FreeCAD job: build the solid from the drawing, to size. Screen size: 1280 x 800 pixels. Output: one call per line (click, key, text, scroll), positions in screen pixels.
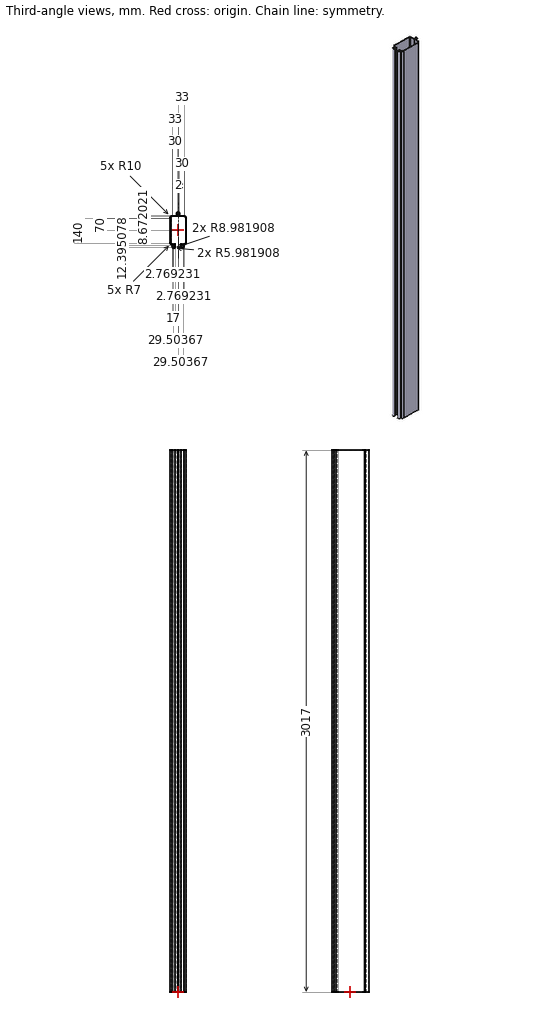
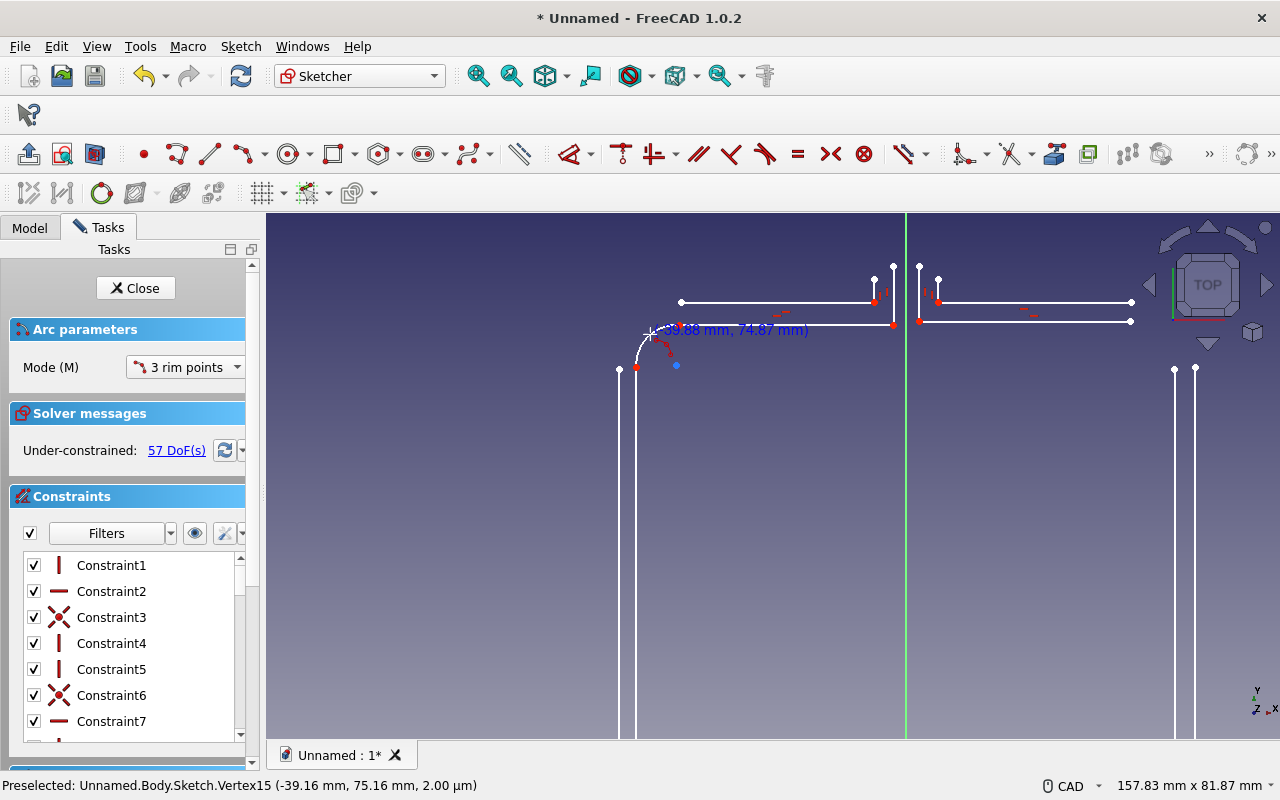
scroll(893, 266, up, 2)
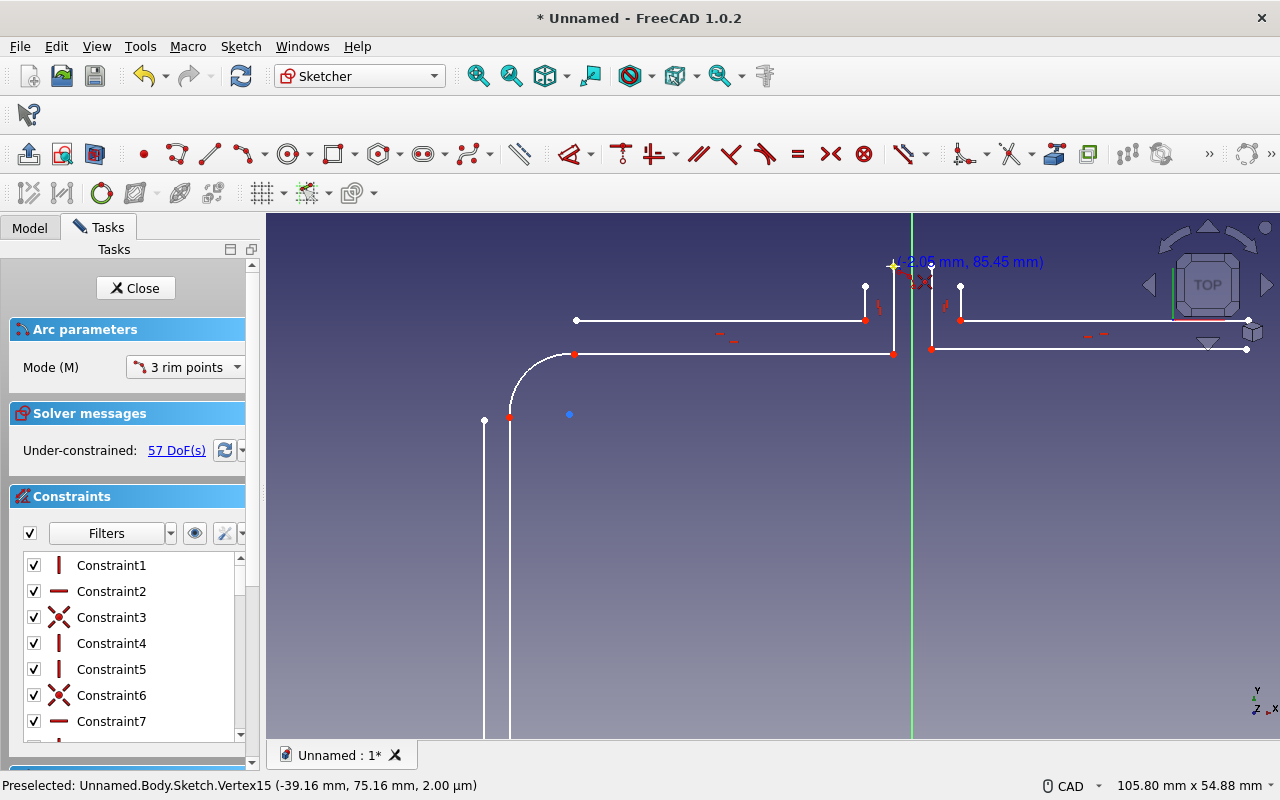
click(894, 266)
click(932, 266)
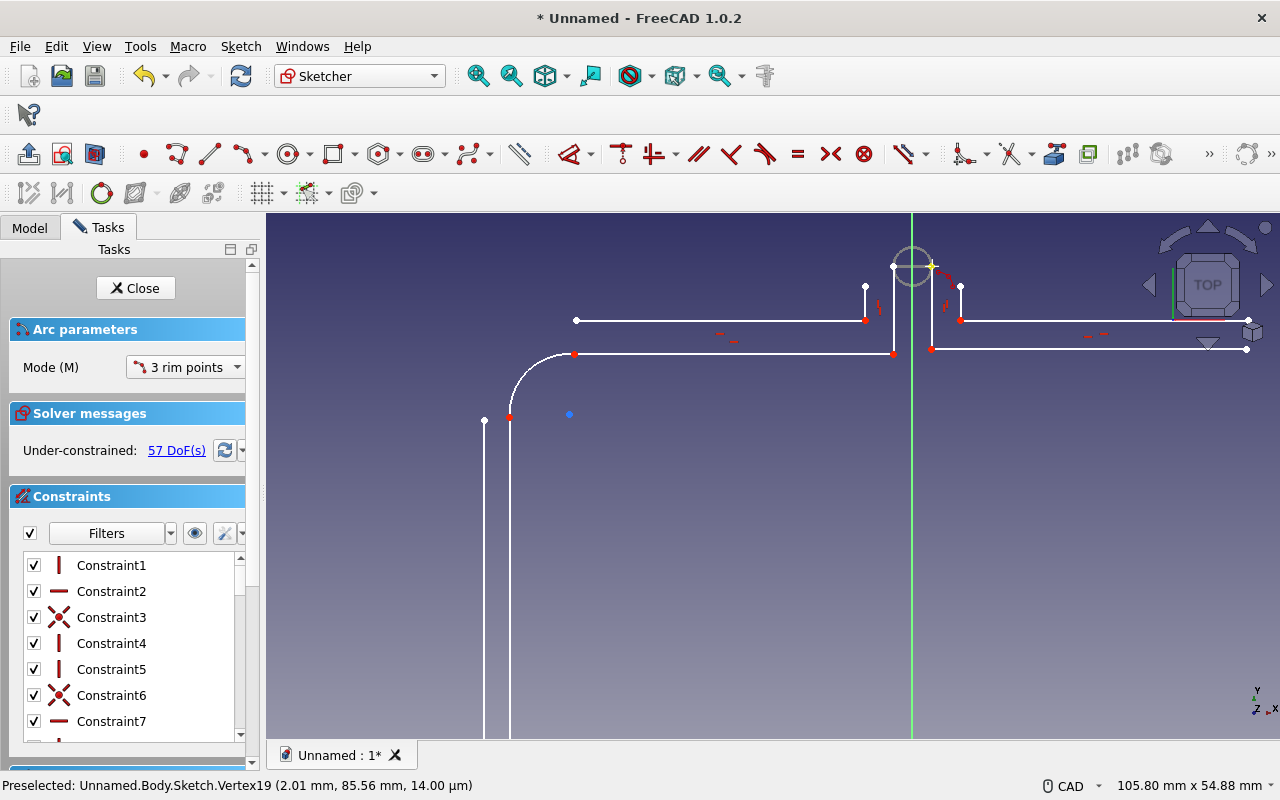
scroll(663, 356, down, 9)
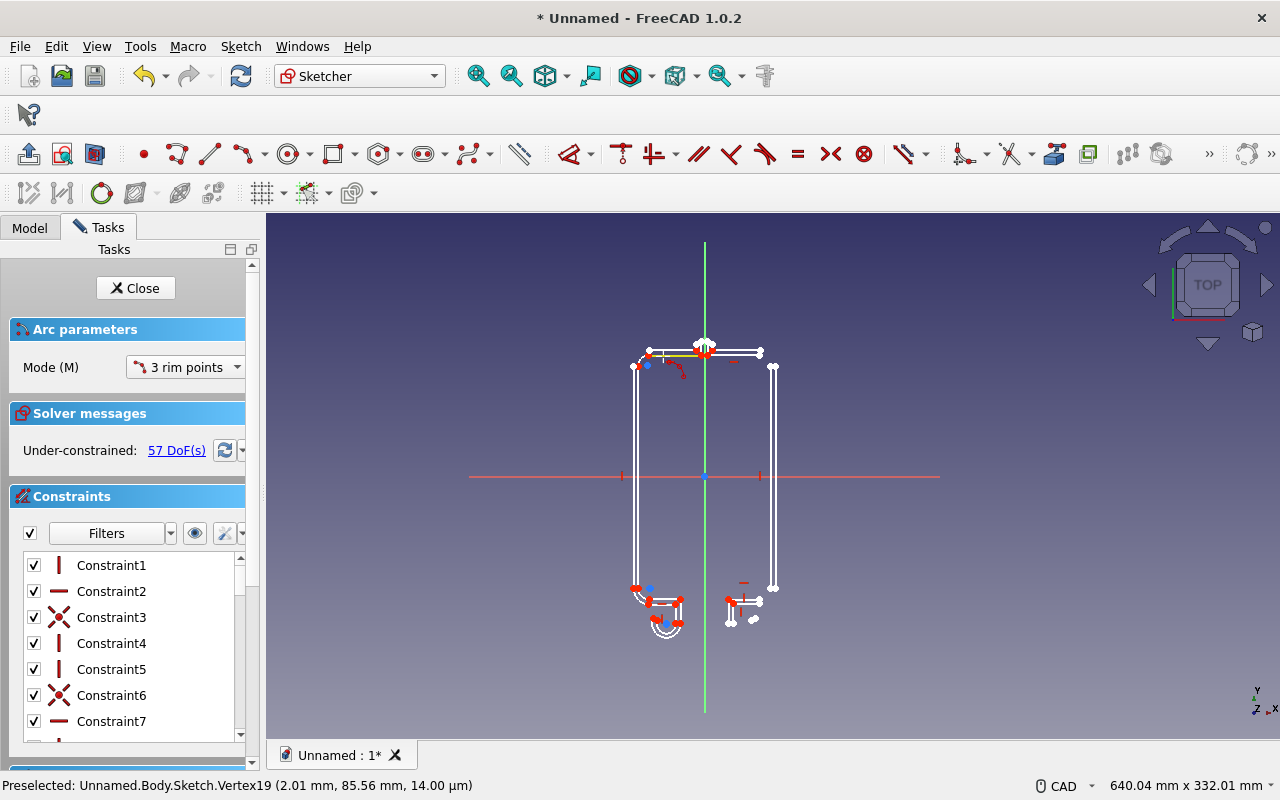
scroll(715, 326, up, 3)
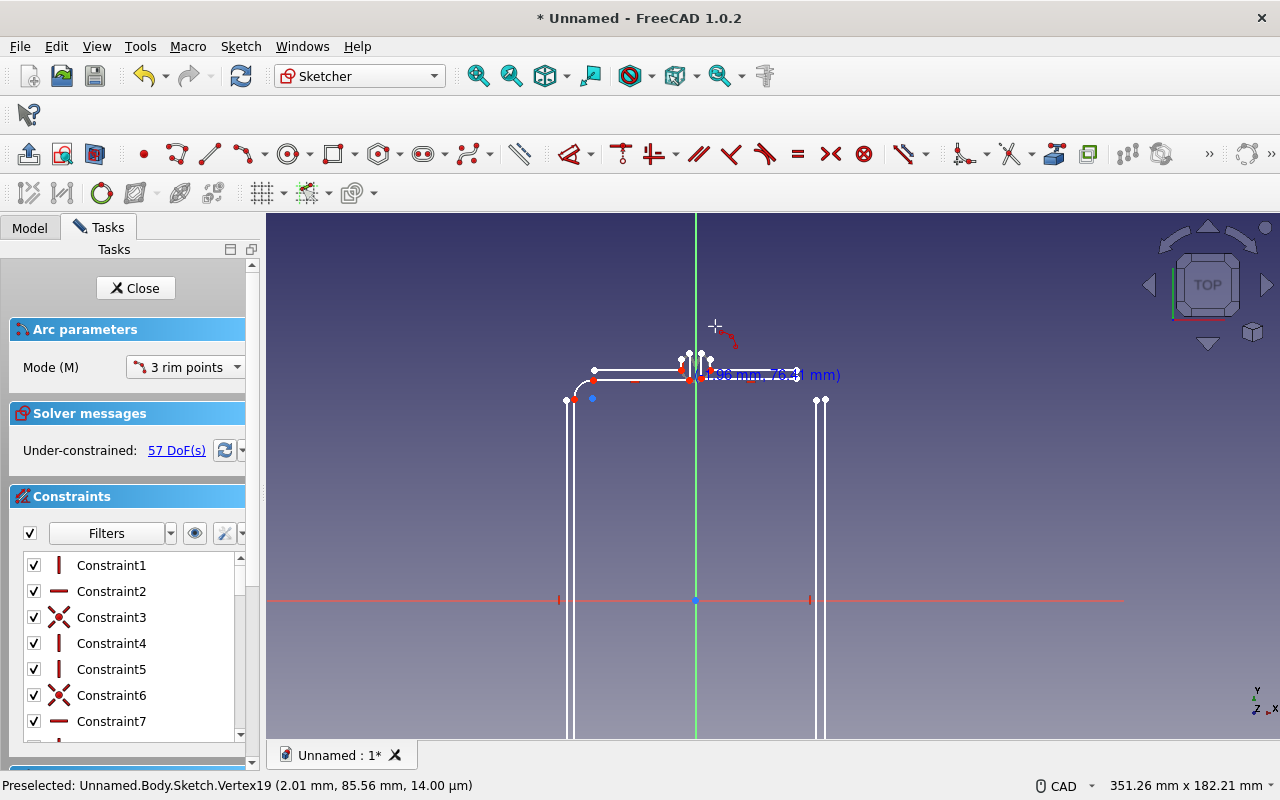
click(714, 326)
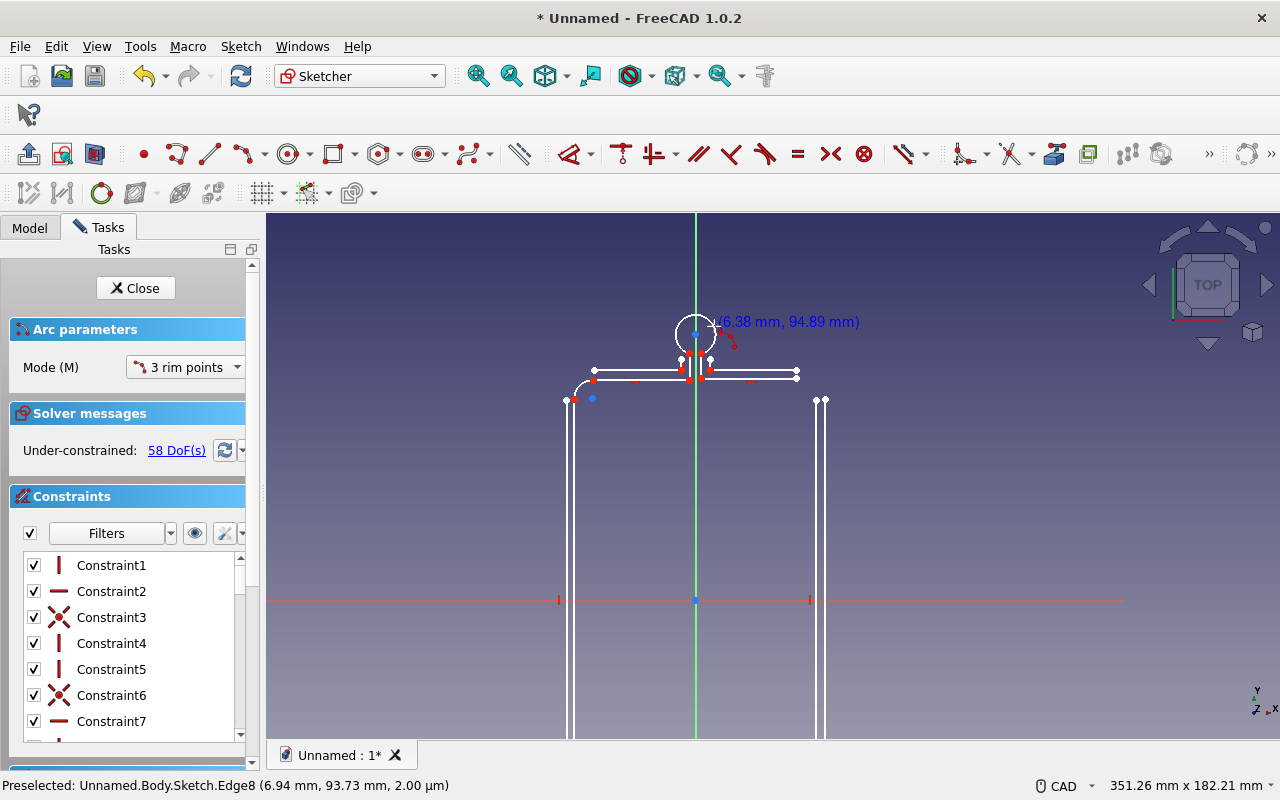
scroll(797, 379, up, 4)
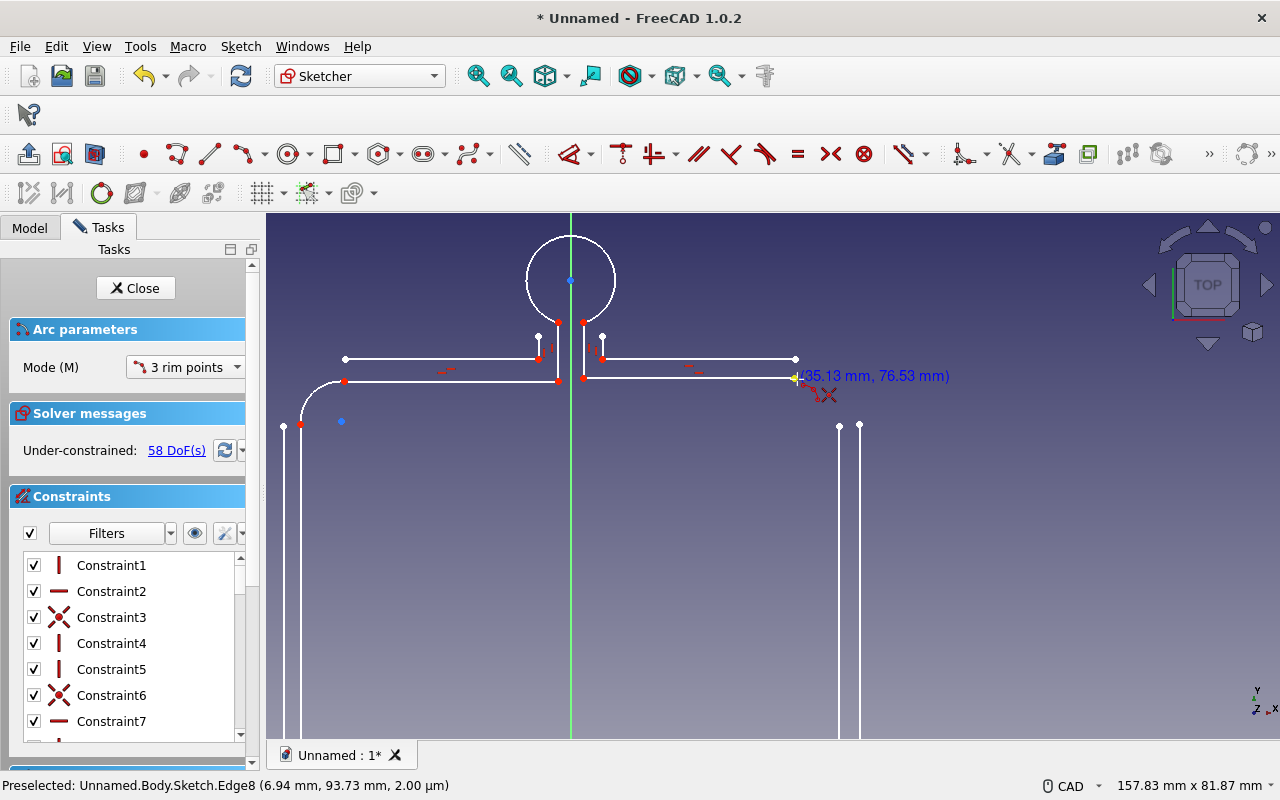
click(795, 378)
click(839, 426)
click(827, 391)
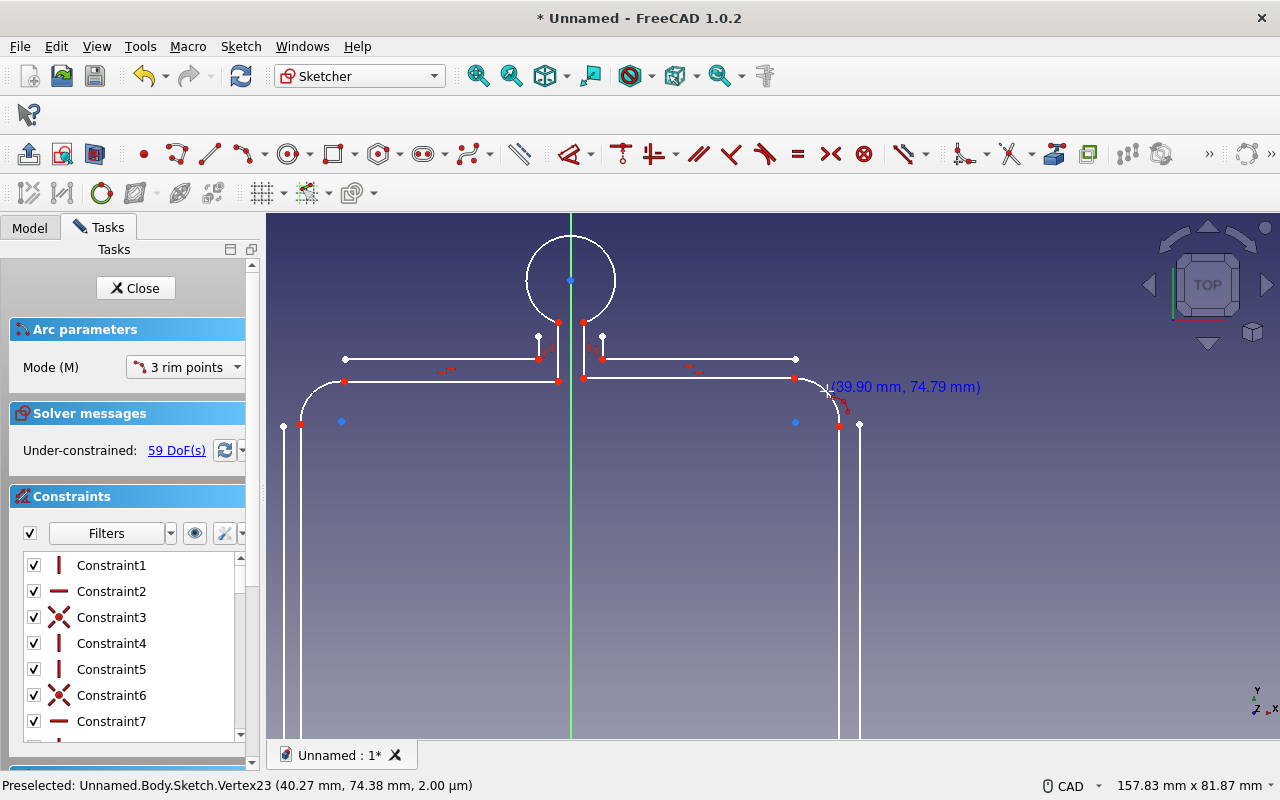
scroll(748, 347, down, 7)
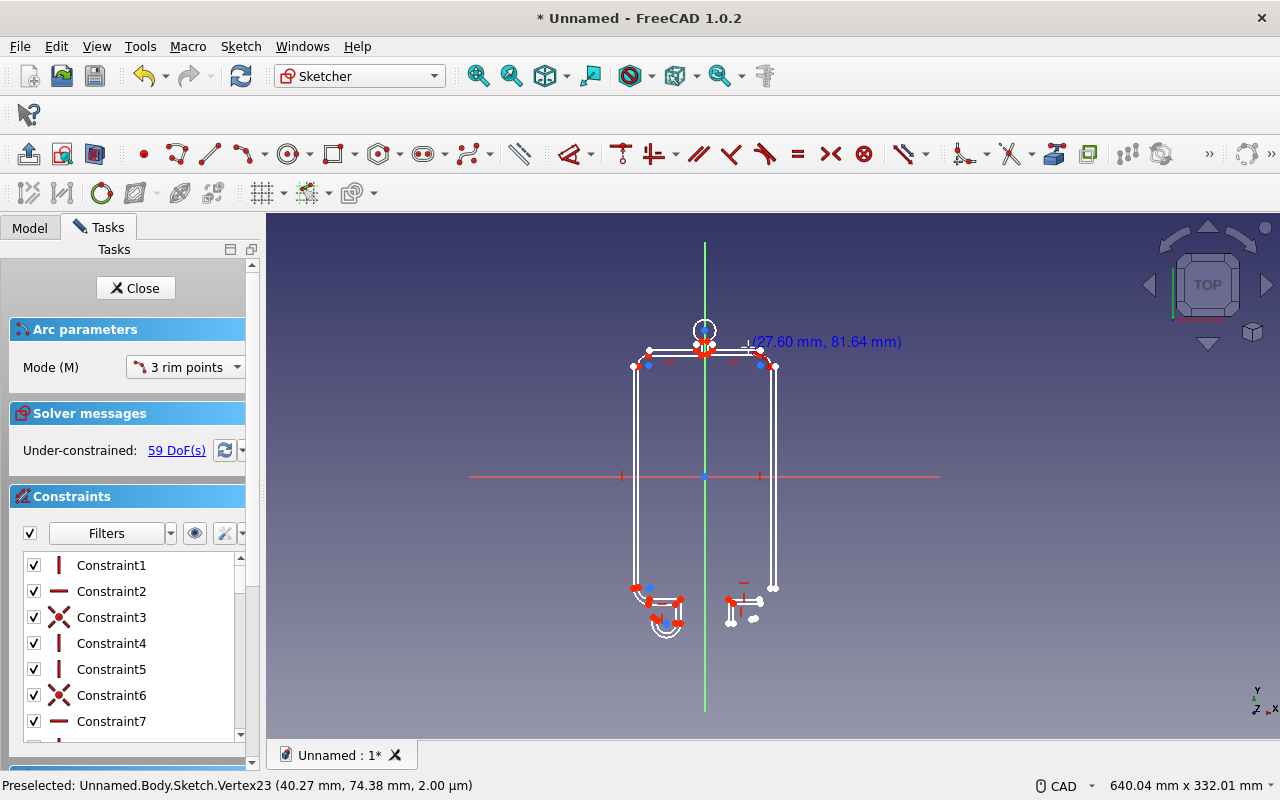
scroll(771, 588, up, 7)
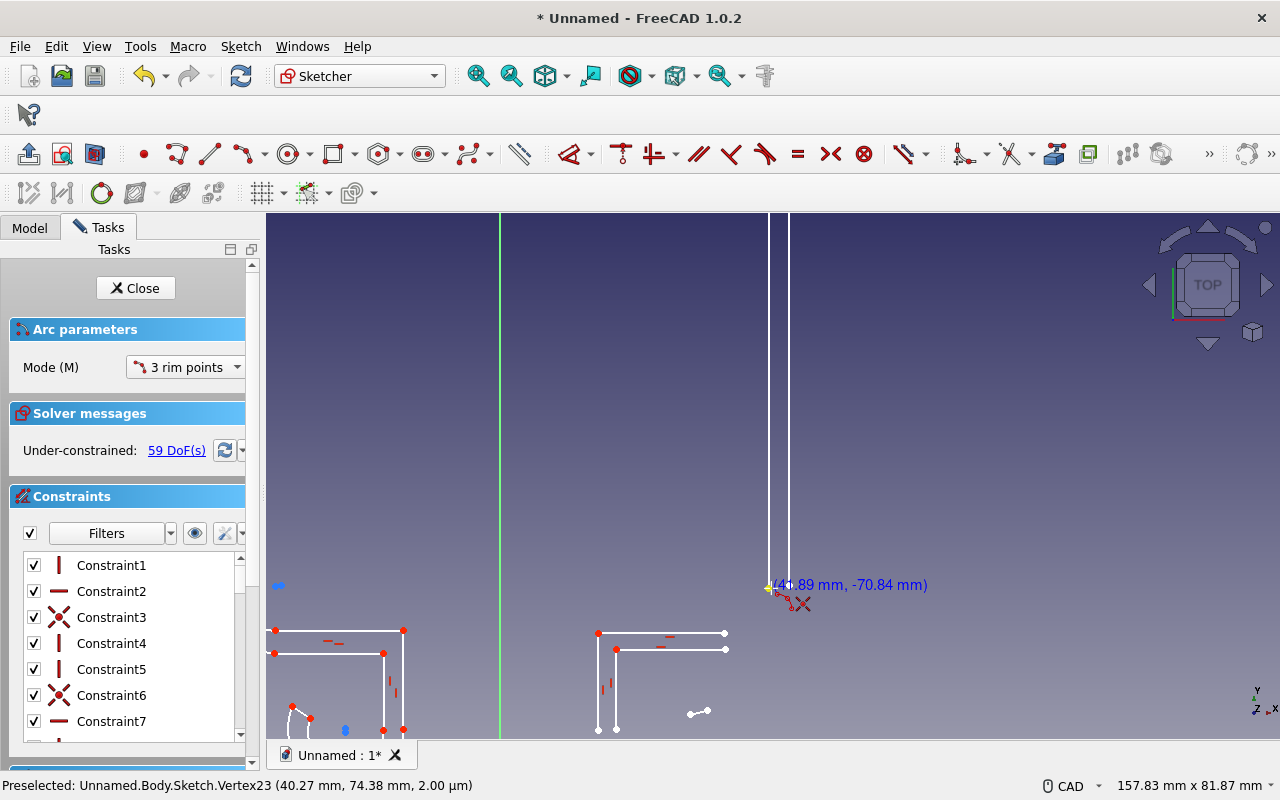
click(769, 589)
click(724, 633)
click(757, 616)